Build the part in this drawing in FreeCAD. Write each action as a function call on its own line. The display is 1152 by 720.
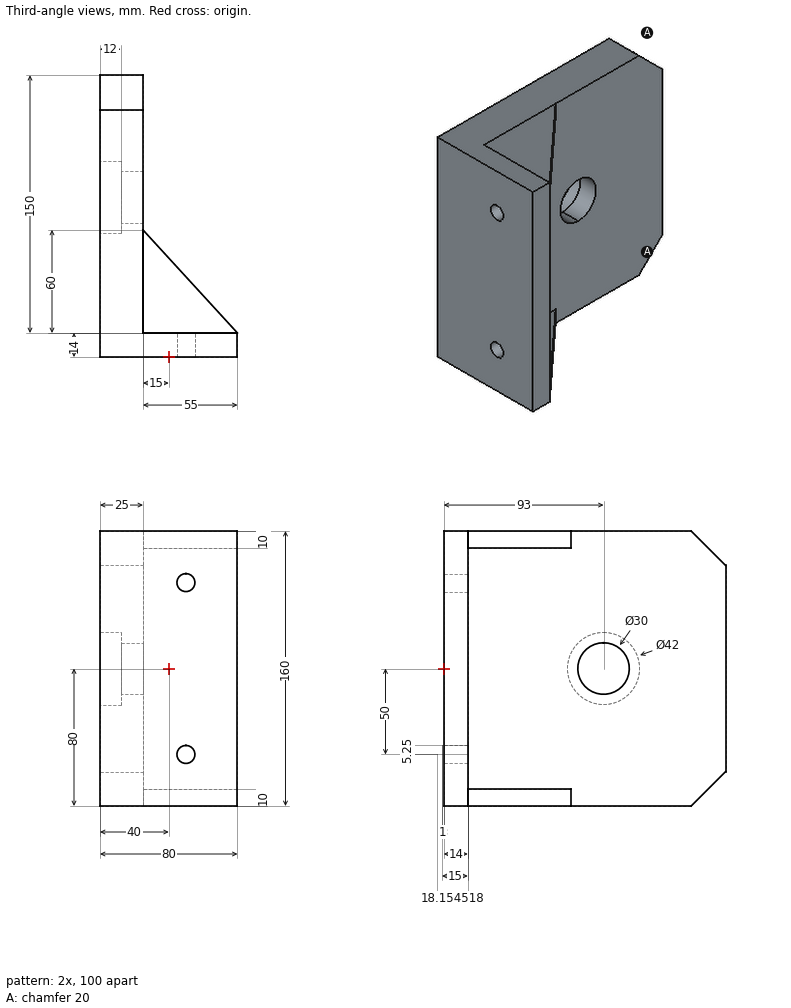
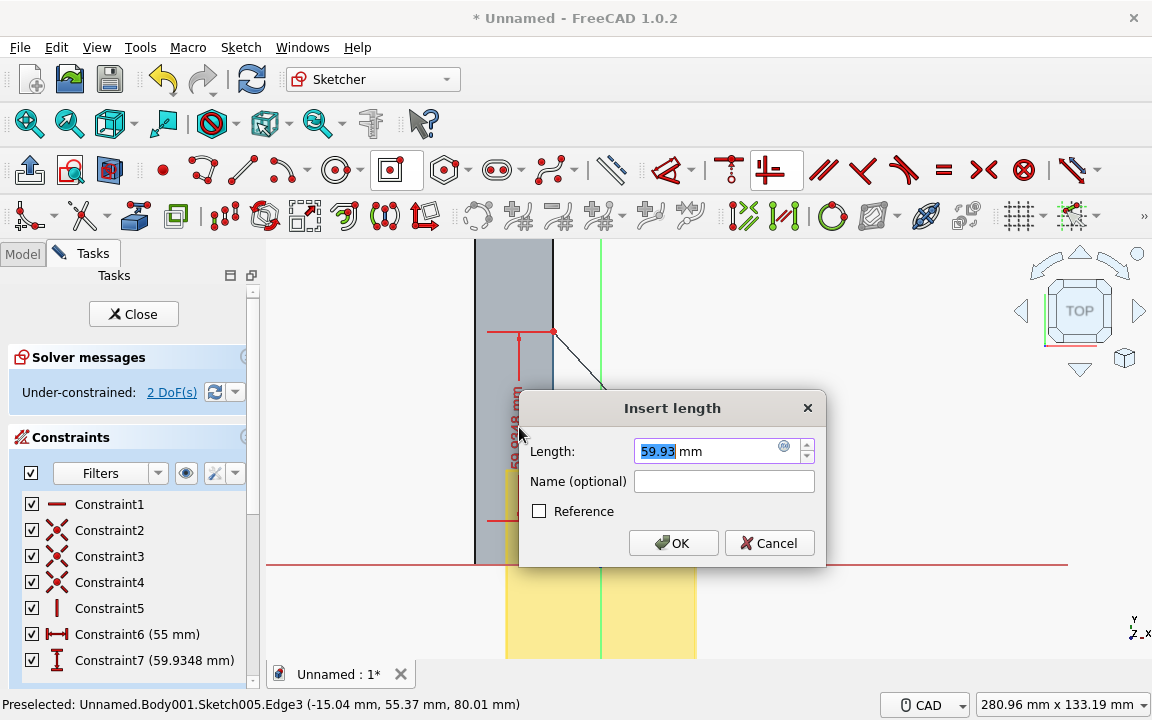
text(60)
key(Return)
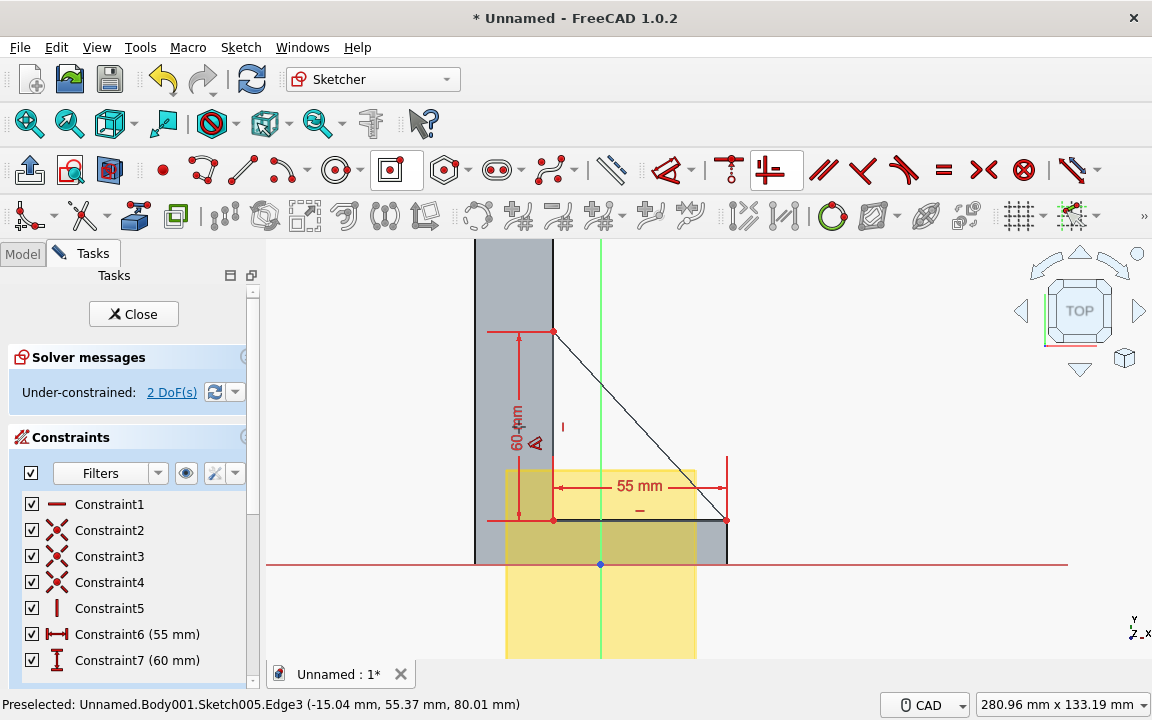
click(553, 521)
click(577, 599)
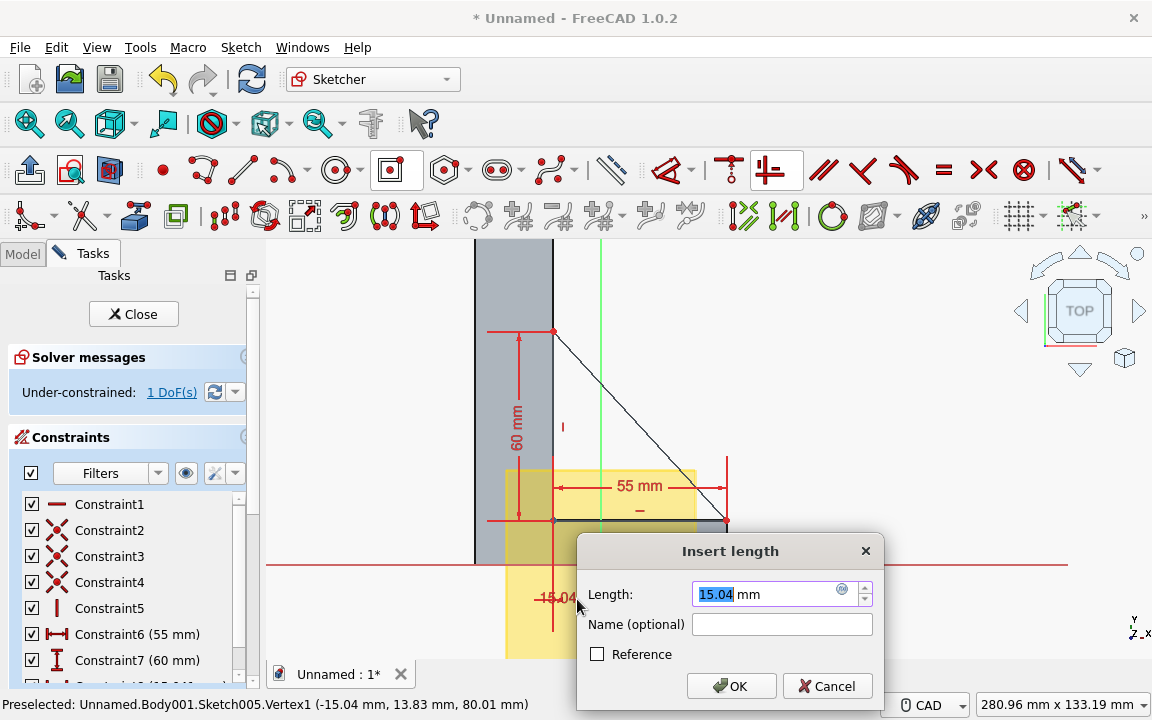
text(15)
key(Return)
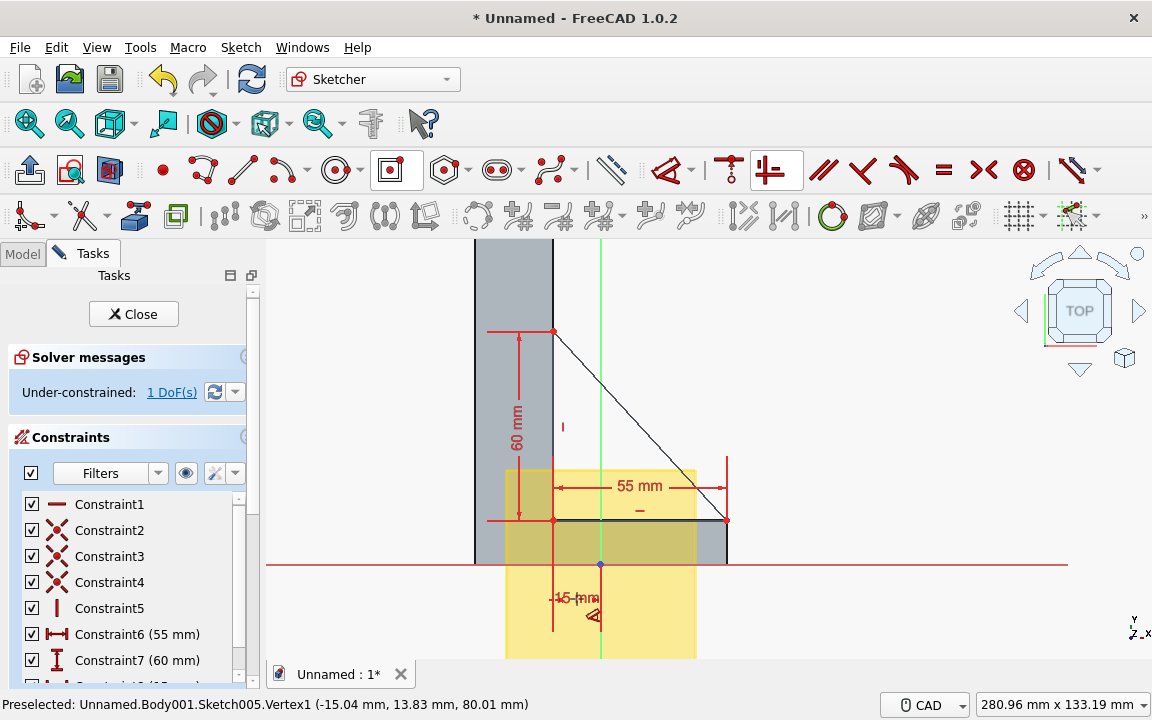
click(553, 521)
click(519, 543)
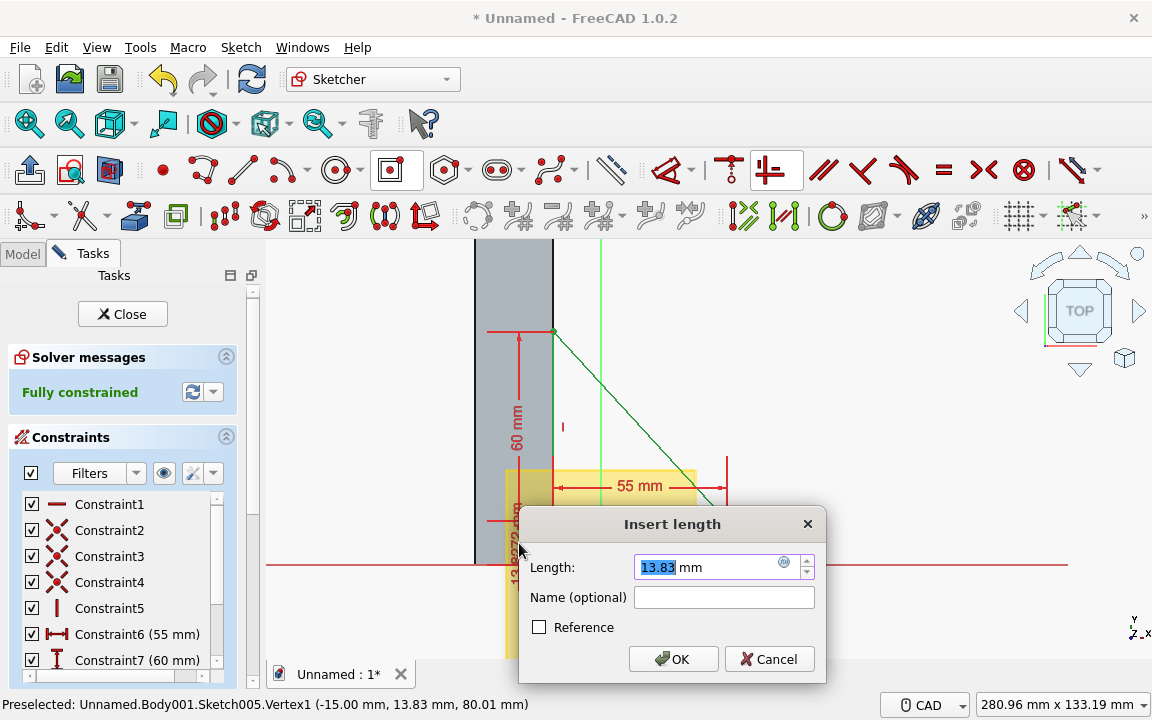
text(14)
key(Return)
key(Escape)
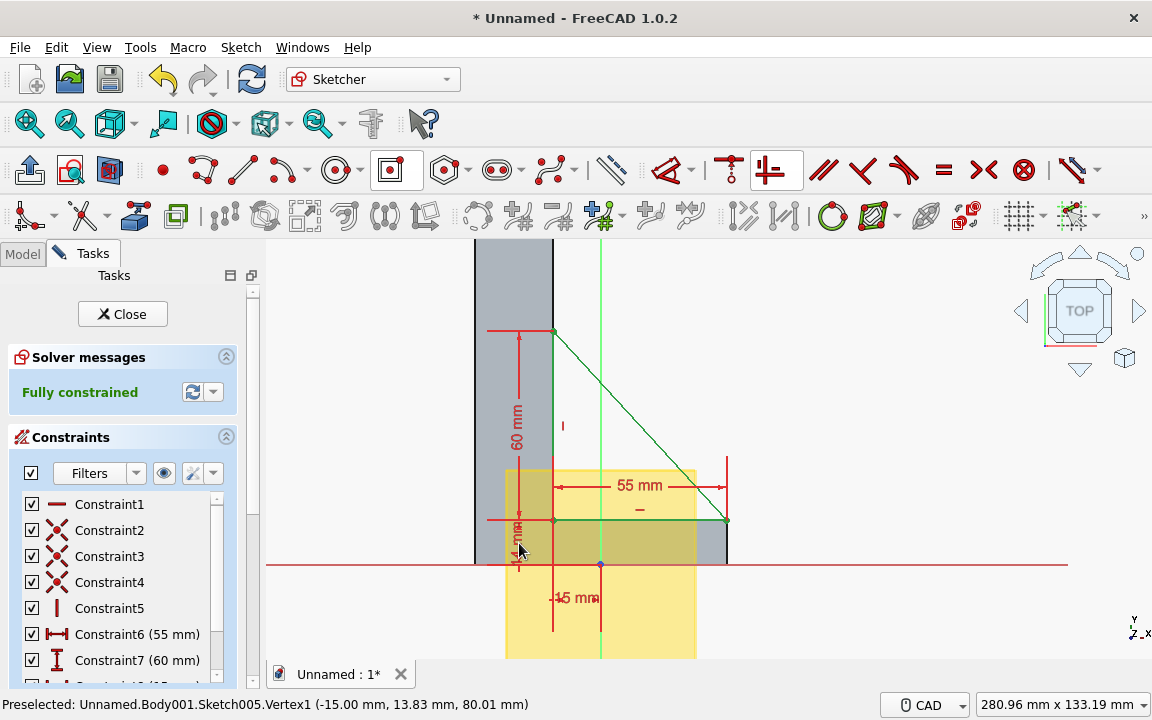
click(123, 314)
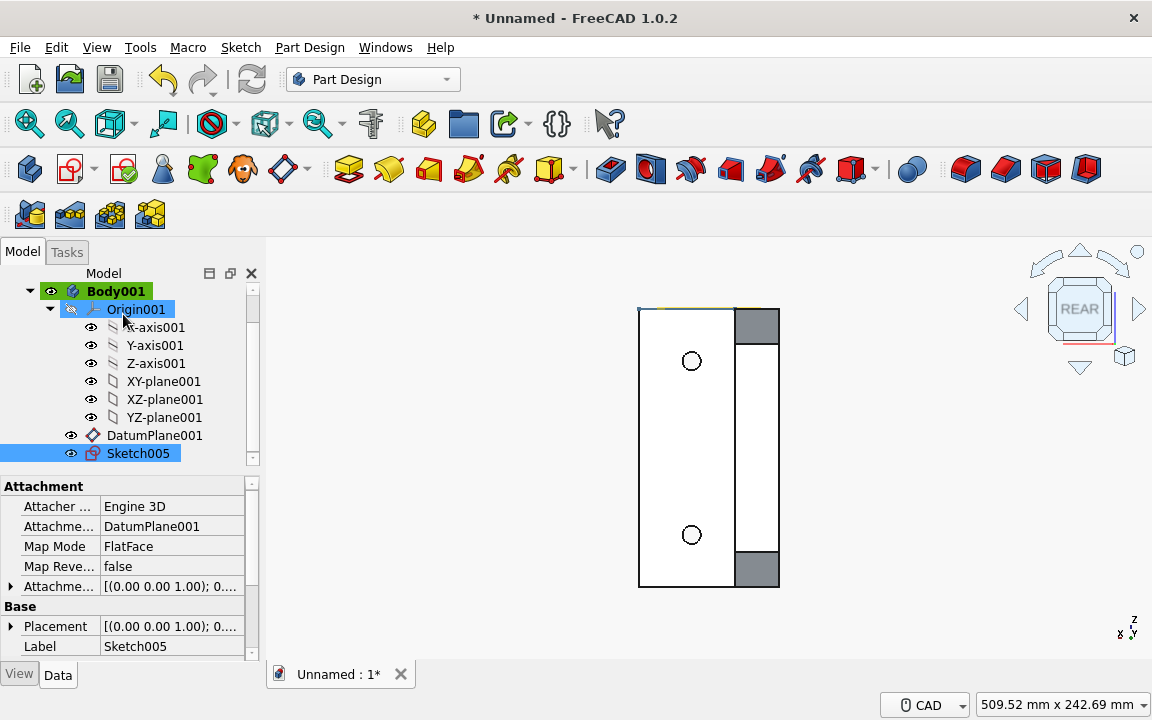
click(350, 170)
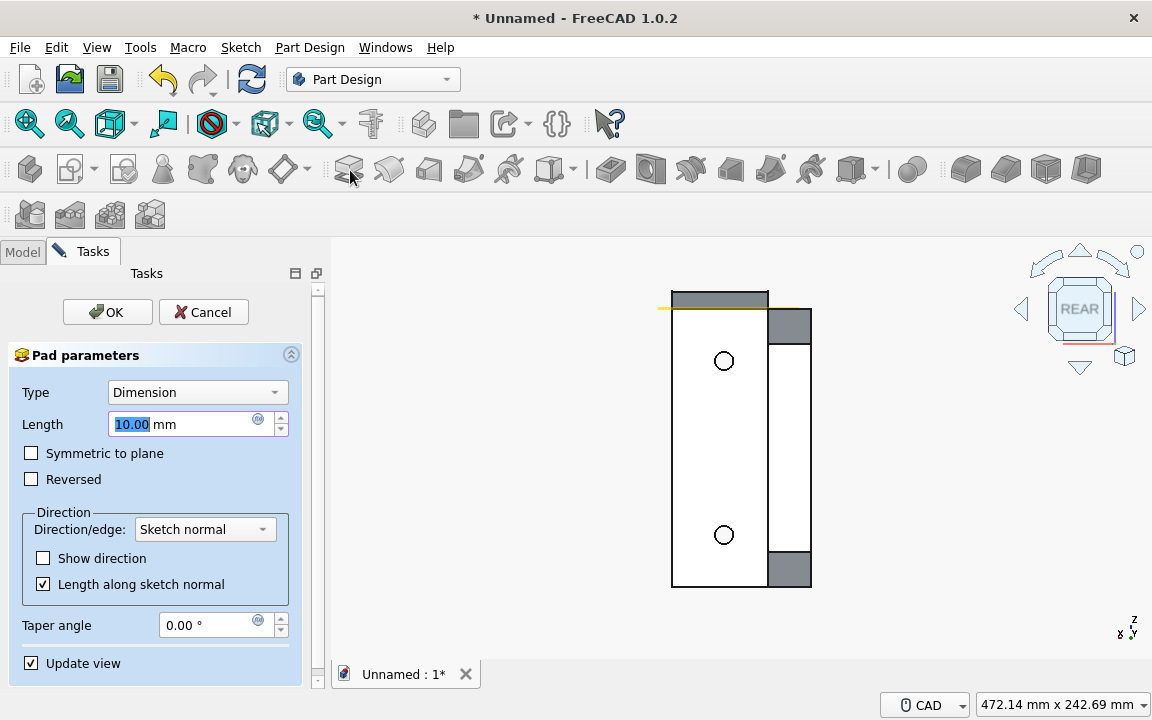
text(10)
key(Tab)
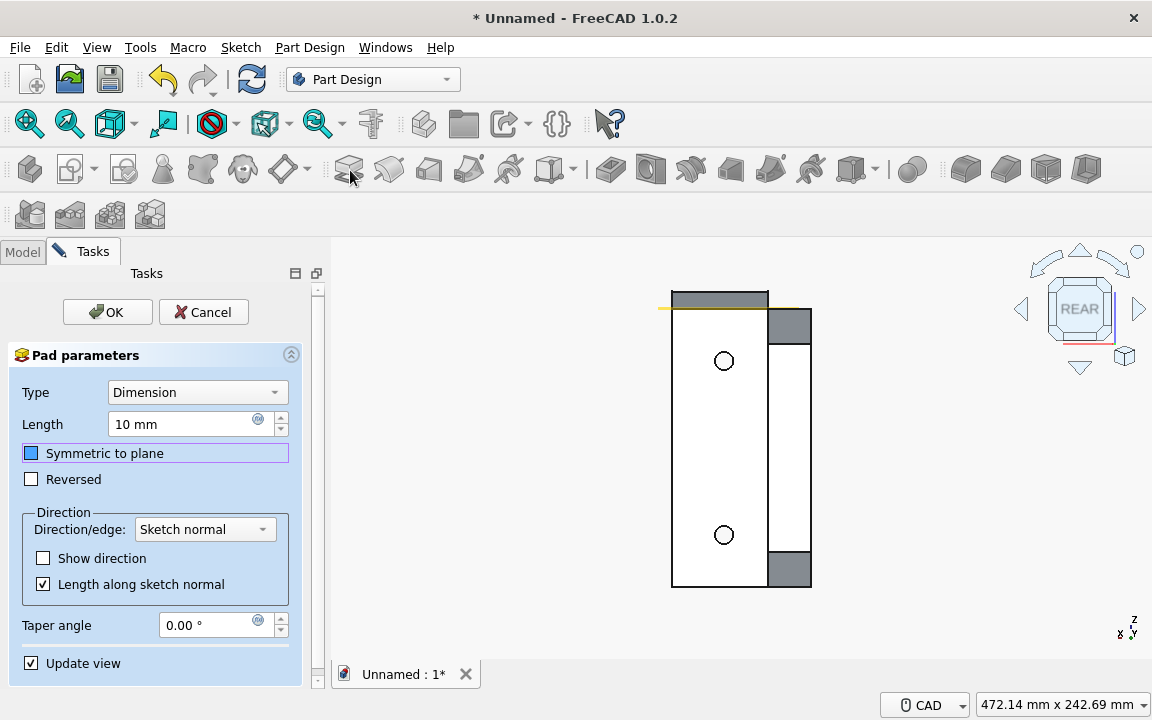
click(30, 479)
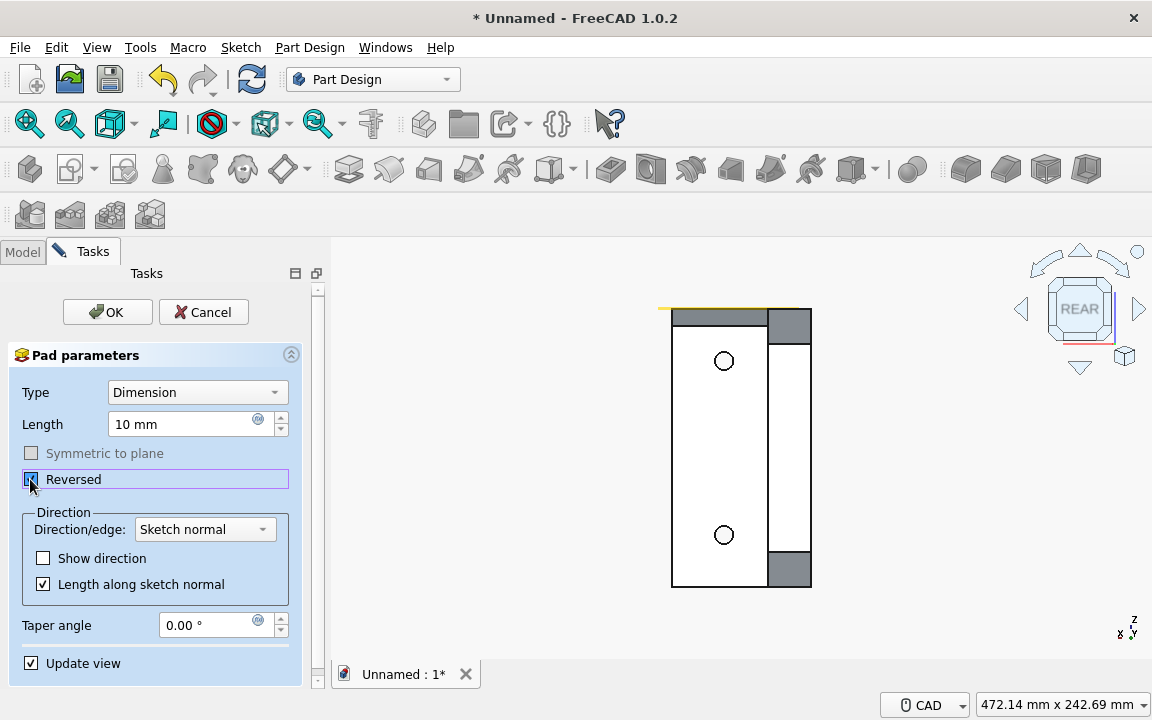
click(108, 312)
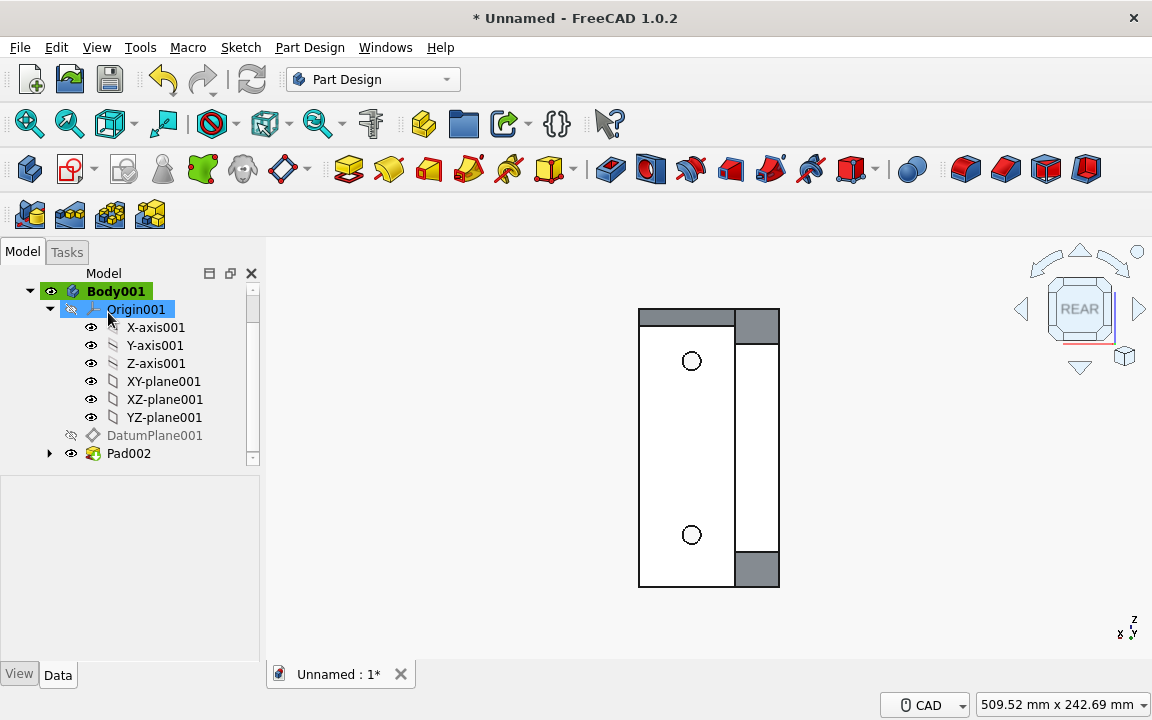
click(30, 124)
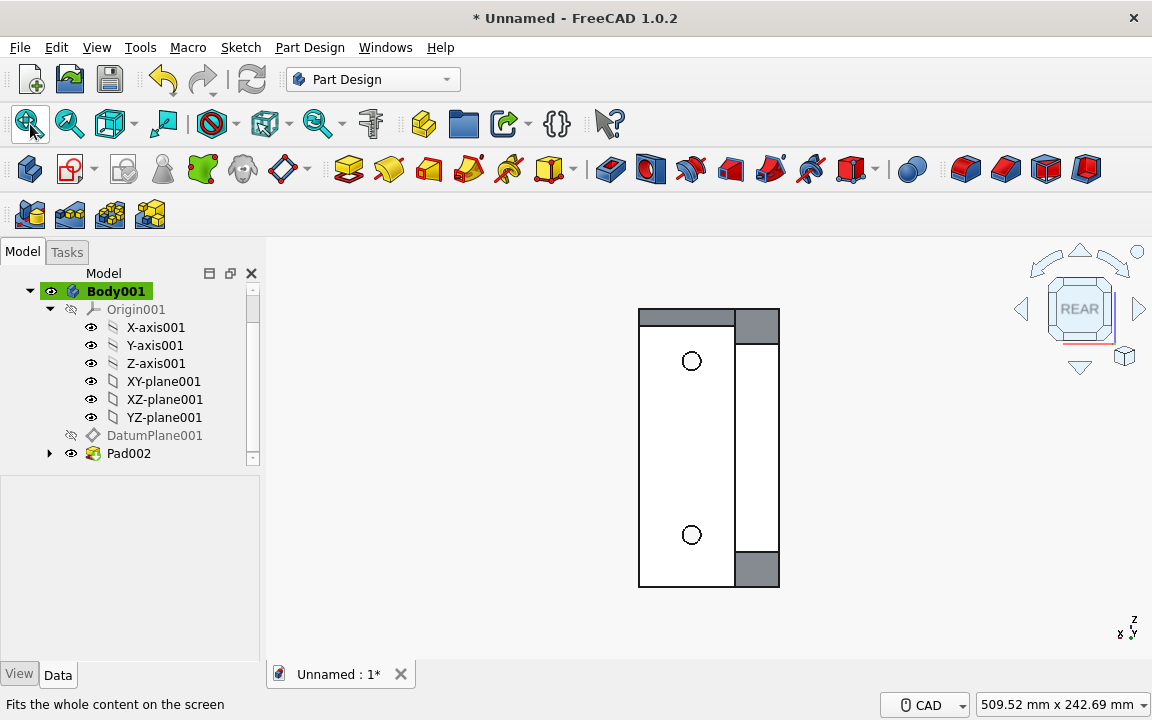
click(30, 170)